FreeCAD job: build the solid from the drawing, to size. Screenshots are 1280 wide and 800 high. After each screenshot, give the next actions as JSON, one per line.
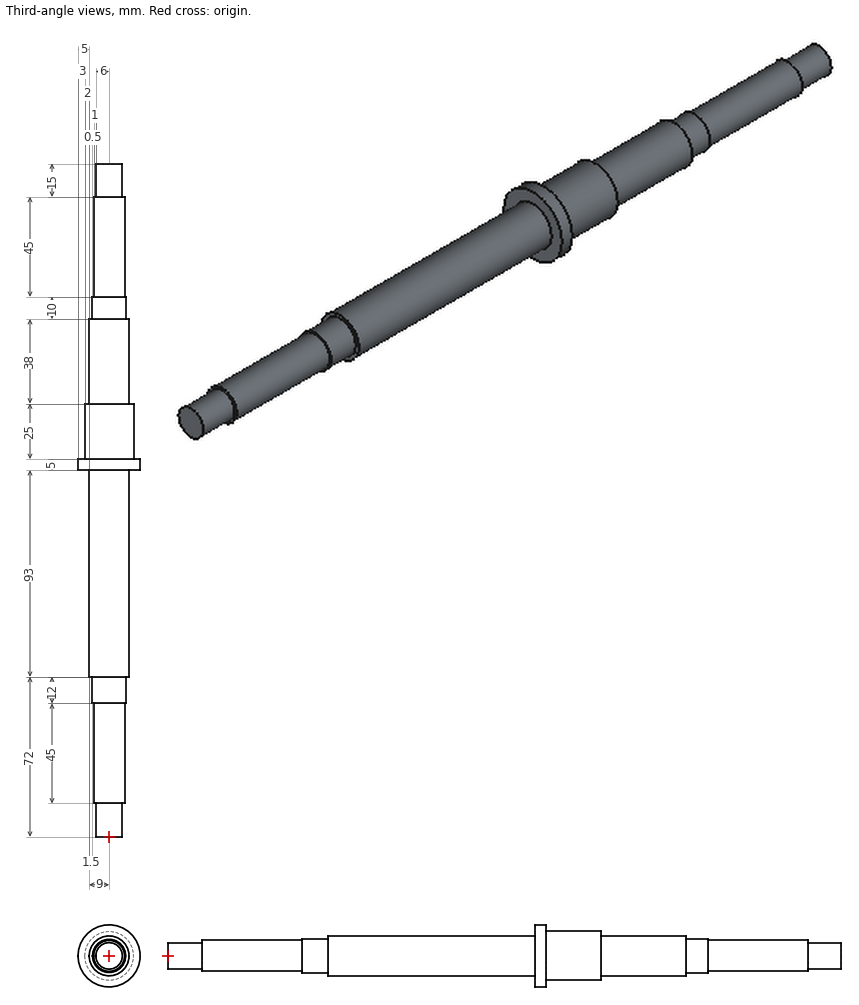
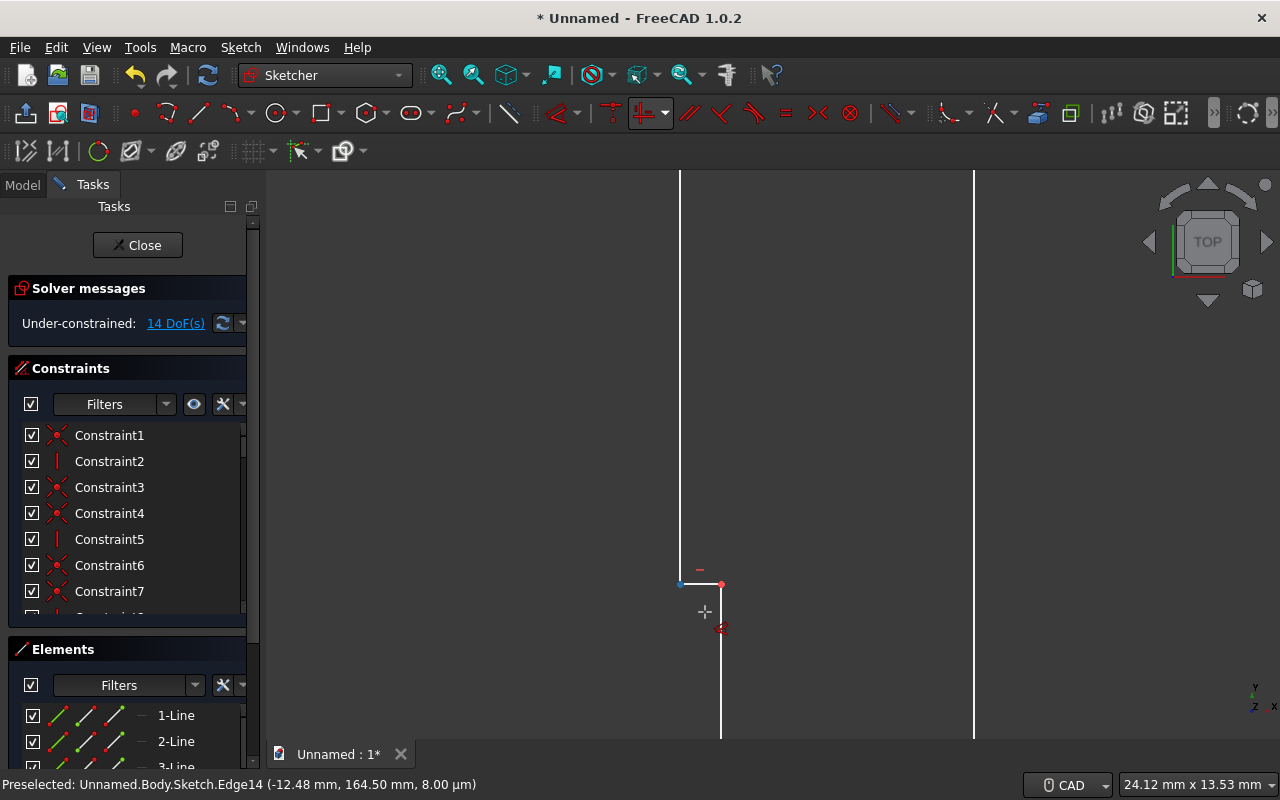
{"action": "left_click", "coordinate": [701, 584]}
{"action": "left_click", "coordinate": [701, 618]}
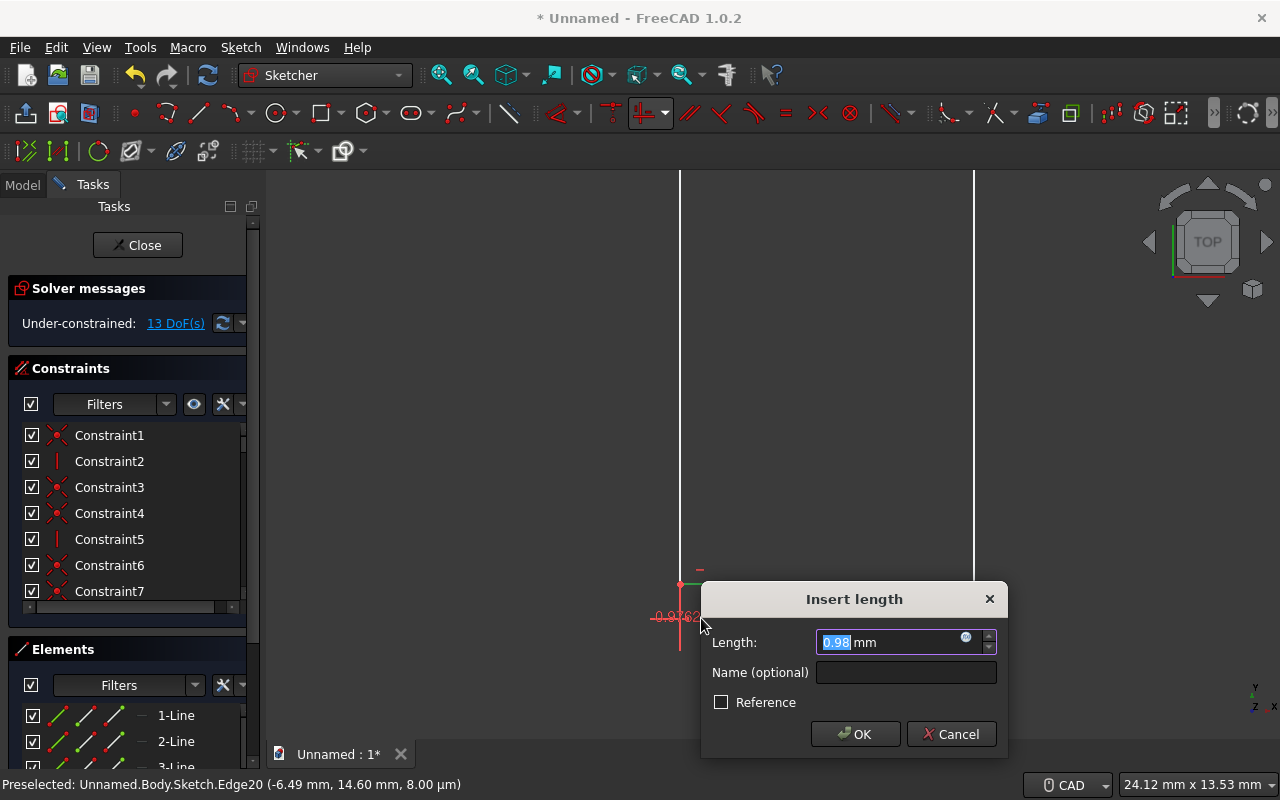
{"action": "type", "text": "1"}
{"action": "key", "text": "Return"}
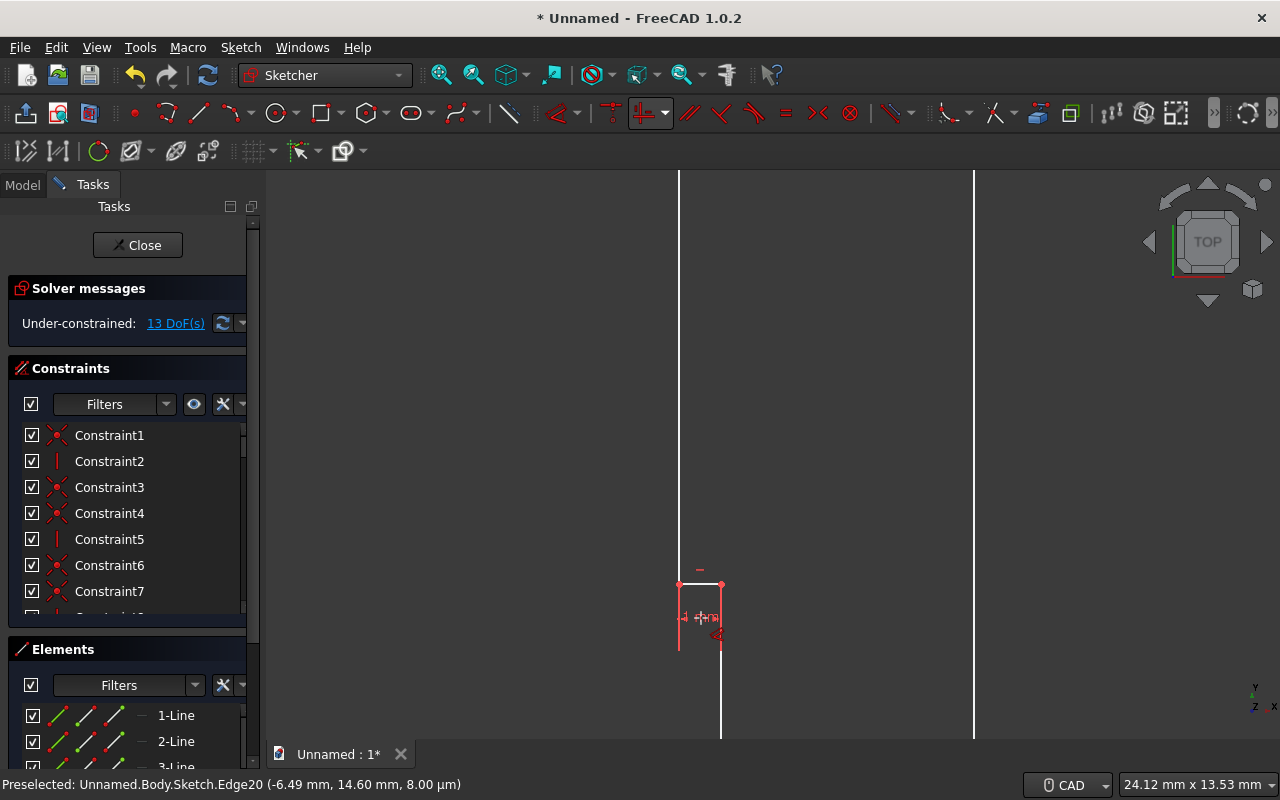
{"action": "scroll", "coordinate": [705, 649], "scroll_direction": "down", "scroll_amount": 17}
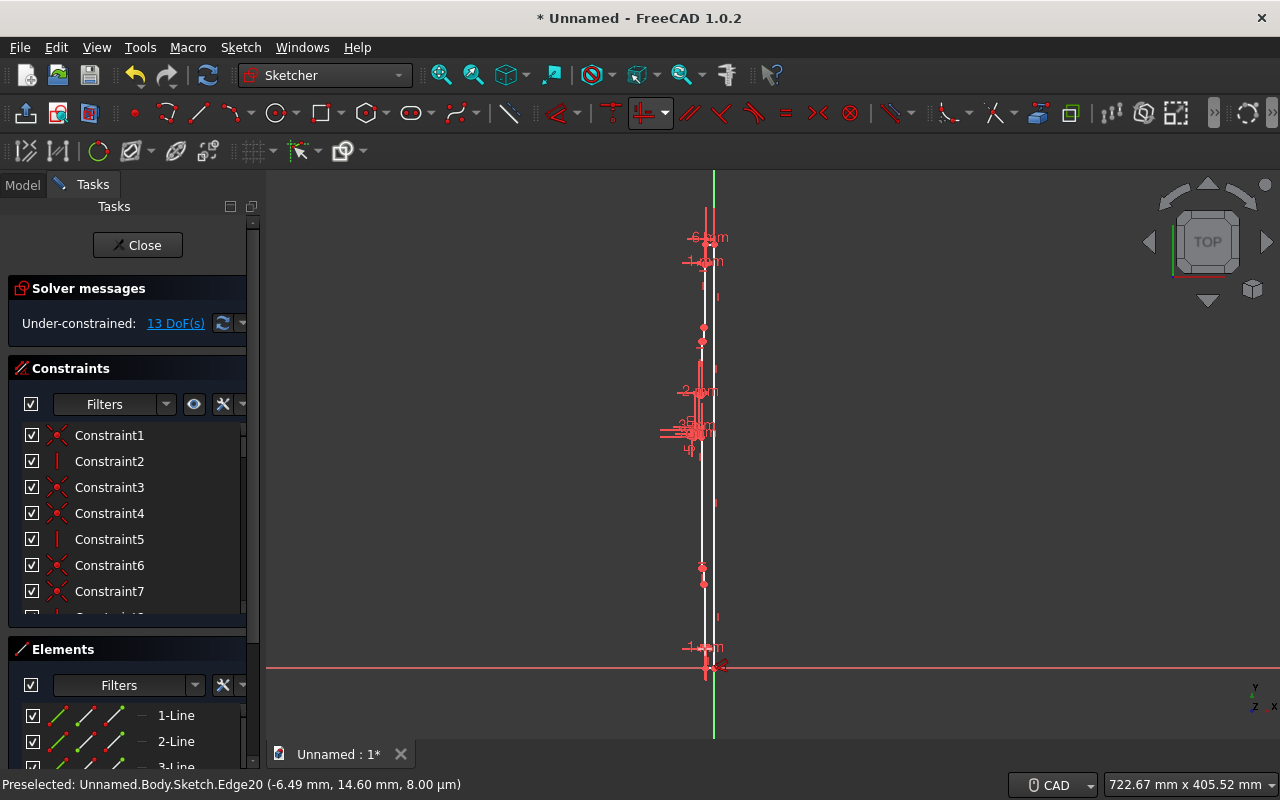
{"action": "scroll", "coordinate": [708, 668], "scroll_direction": "up", "scroll_amount": 9}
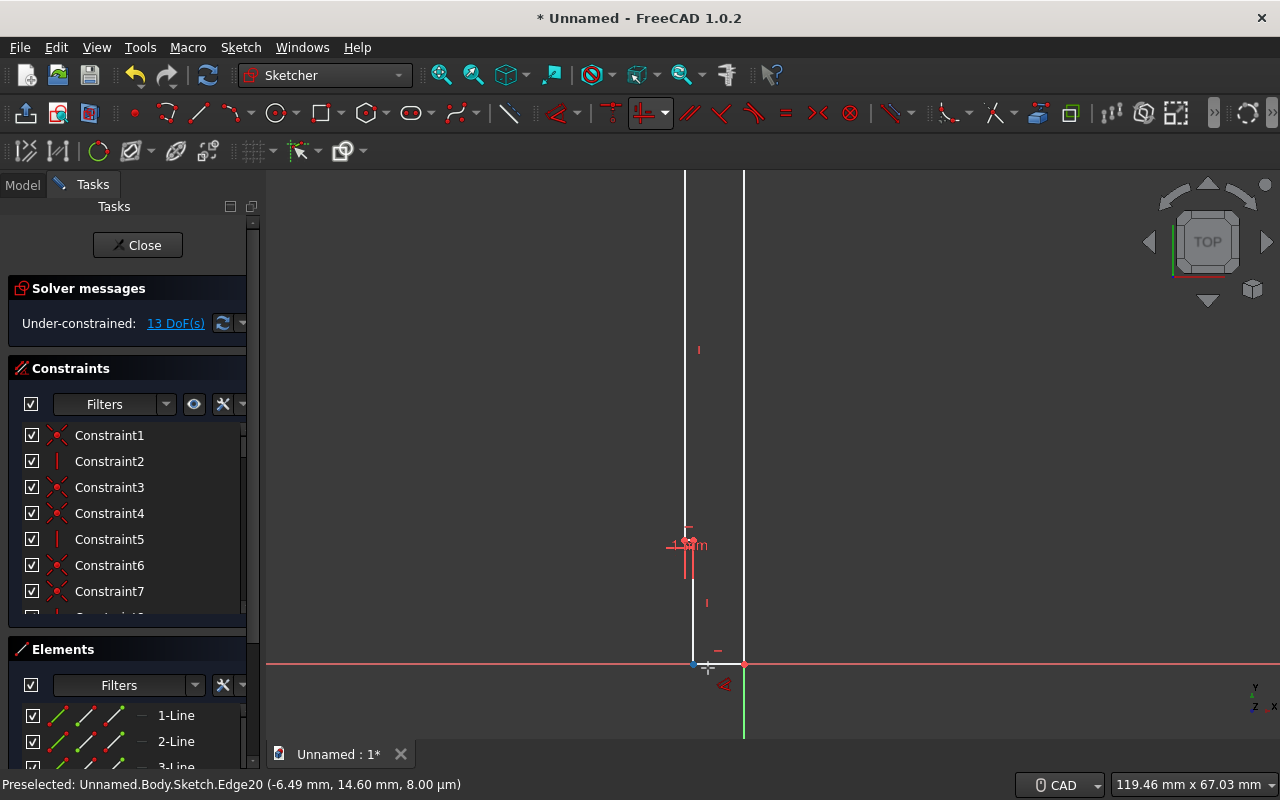
{"action": "left_click", "coordinate": [709, 664]}
{"action": "left_click", "coordinate": [719, 698]}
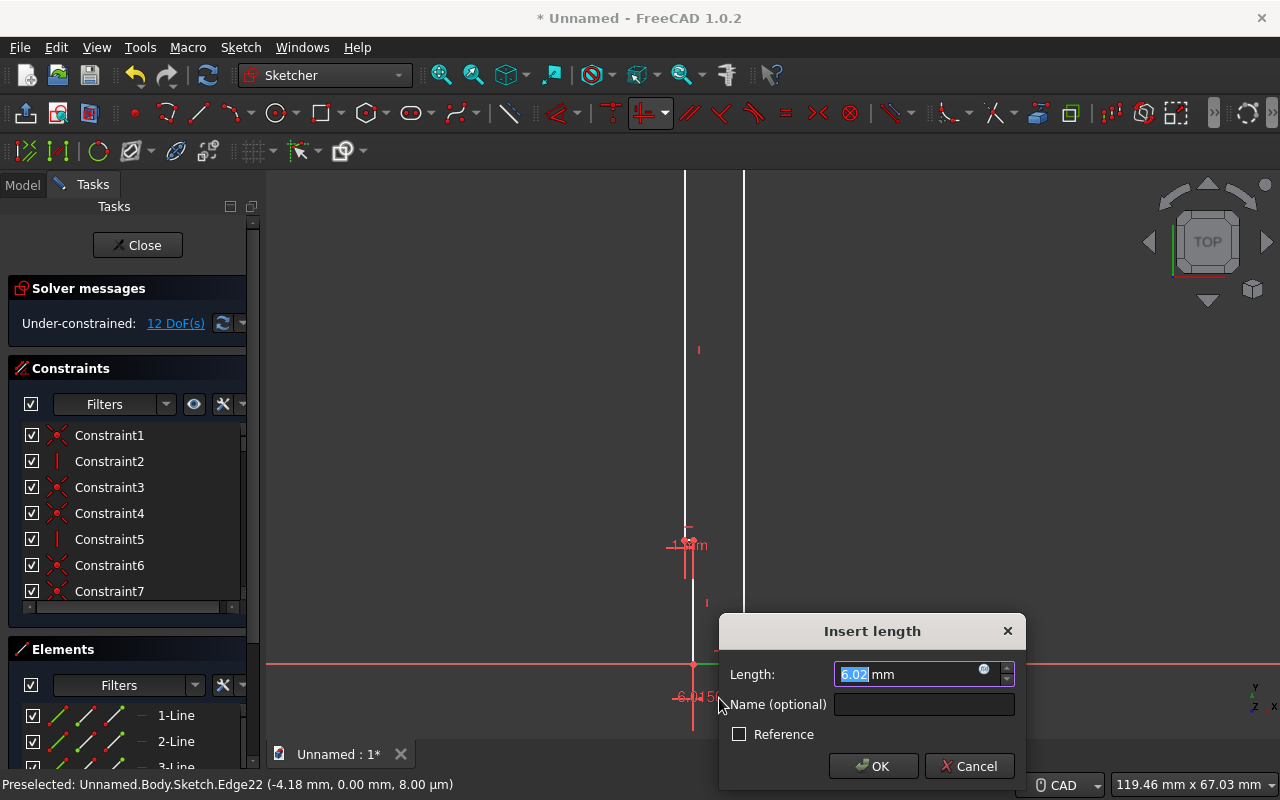
{"action": "type", "text": "6"}
{"action": "key", "text": "Return"}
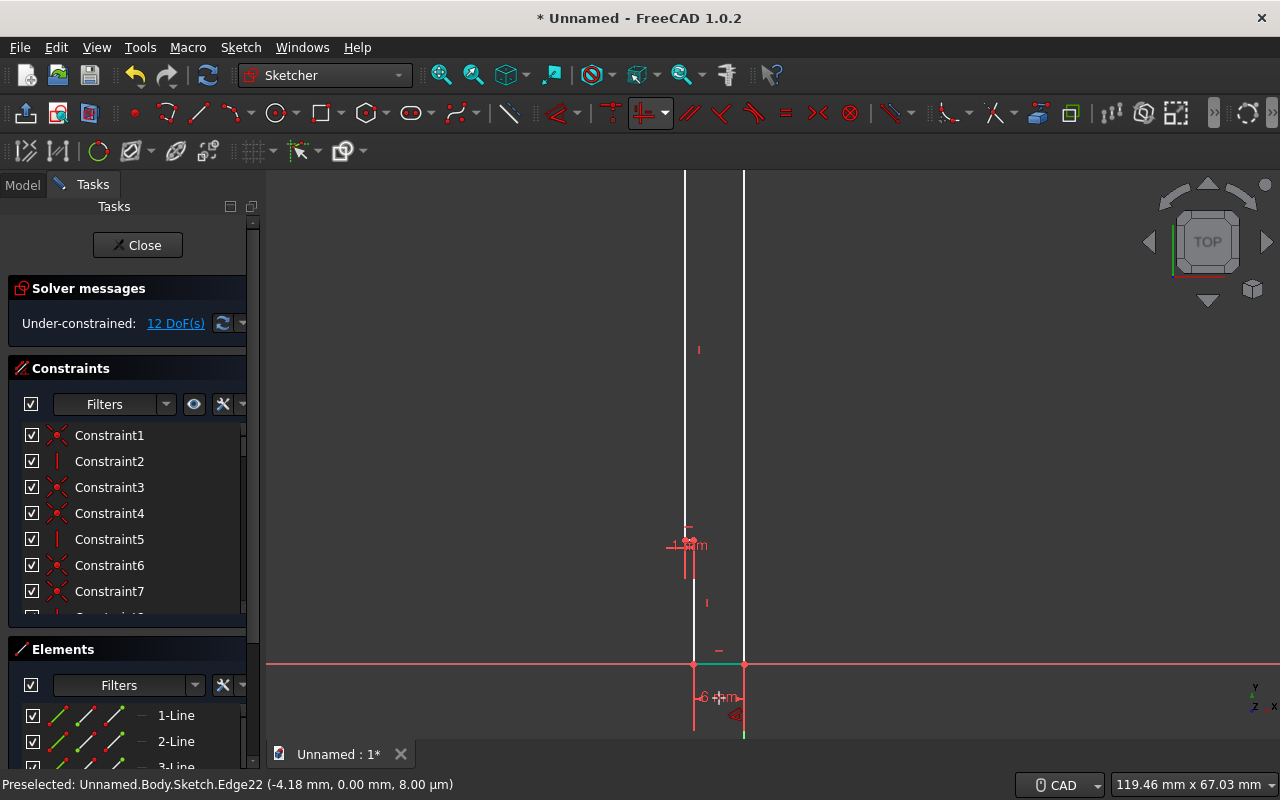
{"action": "scroll", "coordinate": [708, 623], "scroll_direction": "down", "scroll_amount": 10}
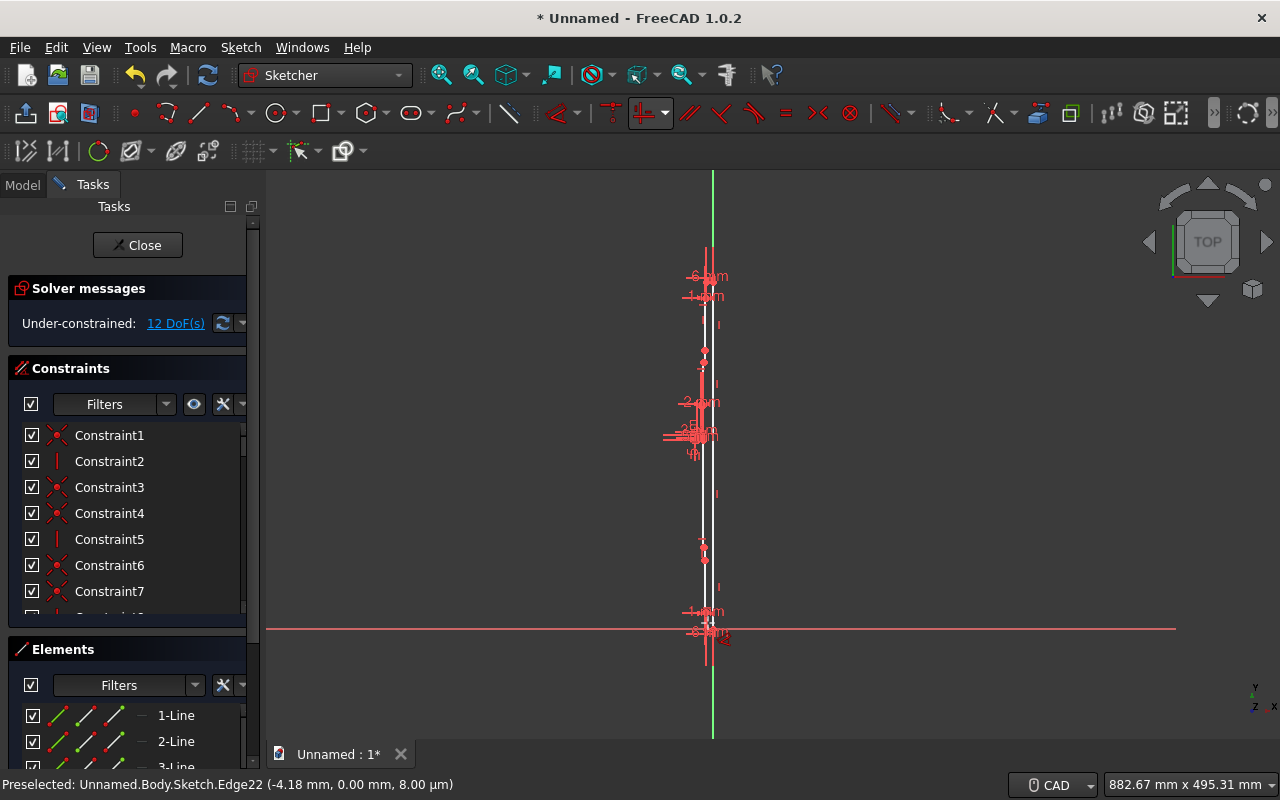
{"action": "scroll", "coordinate": [706, 288], "scroll_direction": "up", "scroll_amount": 6}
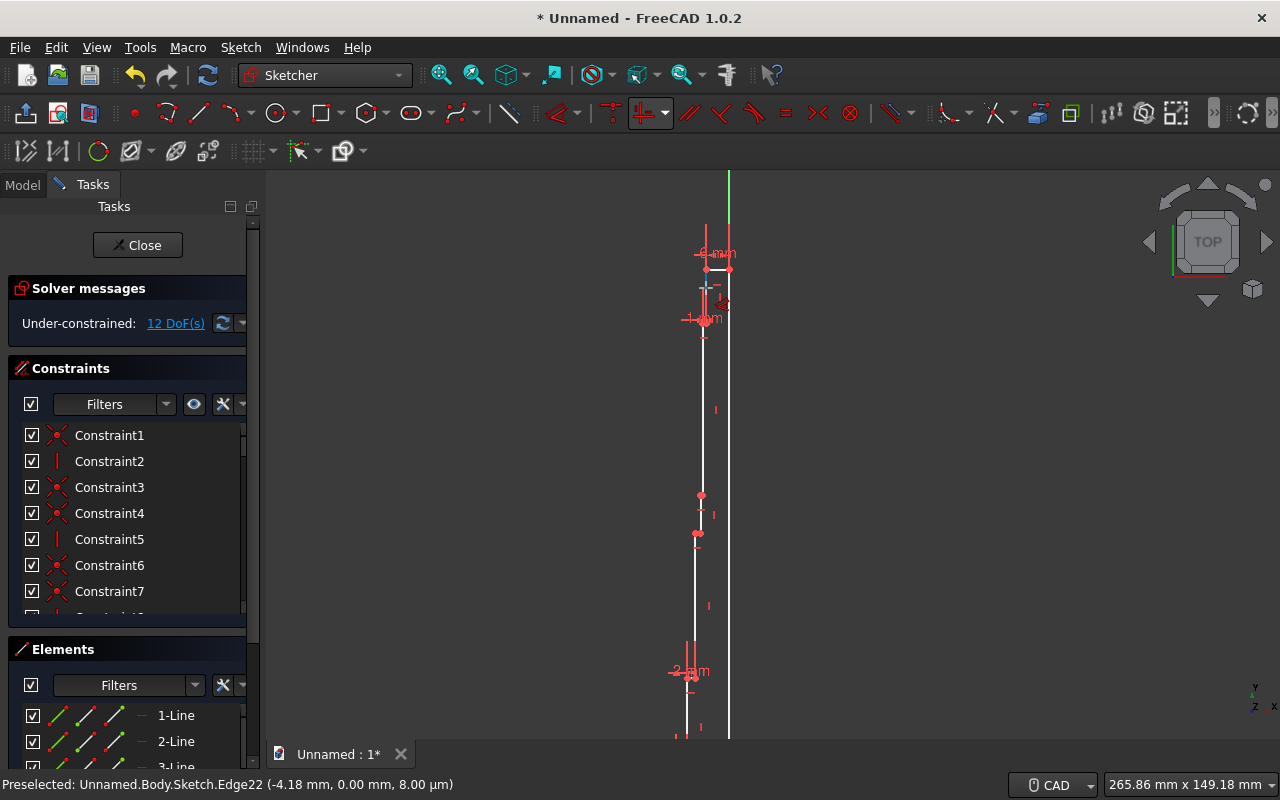
{"action": "left_click", "coordinate": [706, 286]}
{"action": "left_click", "coordinate": [672, 297]}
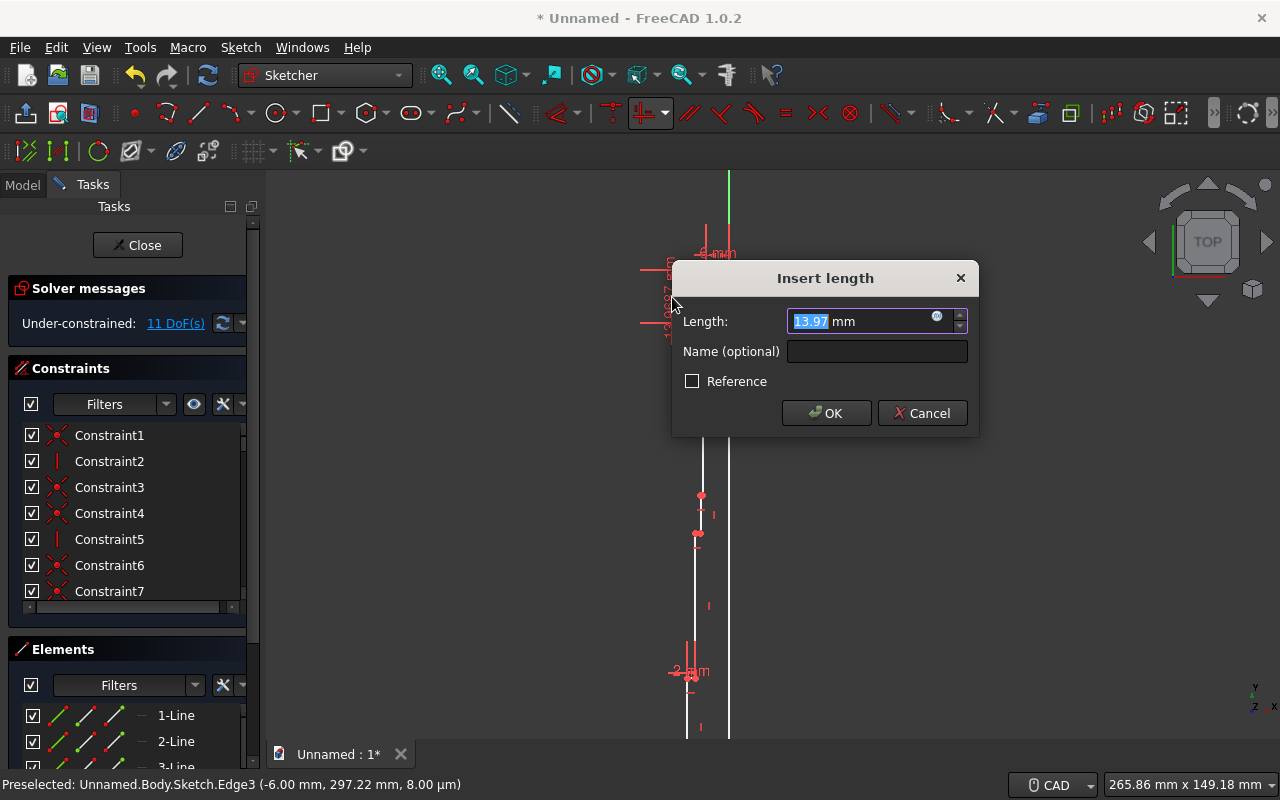
{"action": "type", "text": "15"}
{"action": "key", "text": "Return"}